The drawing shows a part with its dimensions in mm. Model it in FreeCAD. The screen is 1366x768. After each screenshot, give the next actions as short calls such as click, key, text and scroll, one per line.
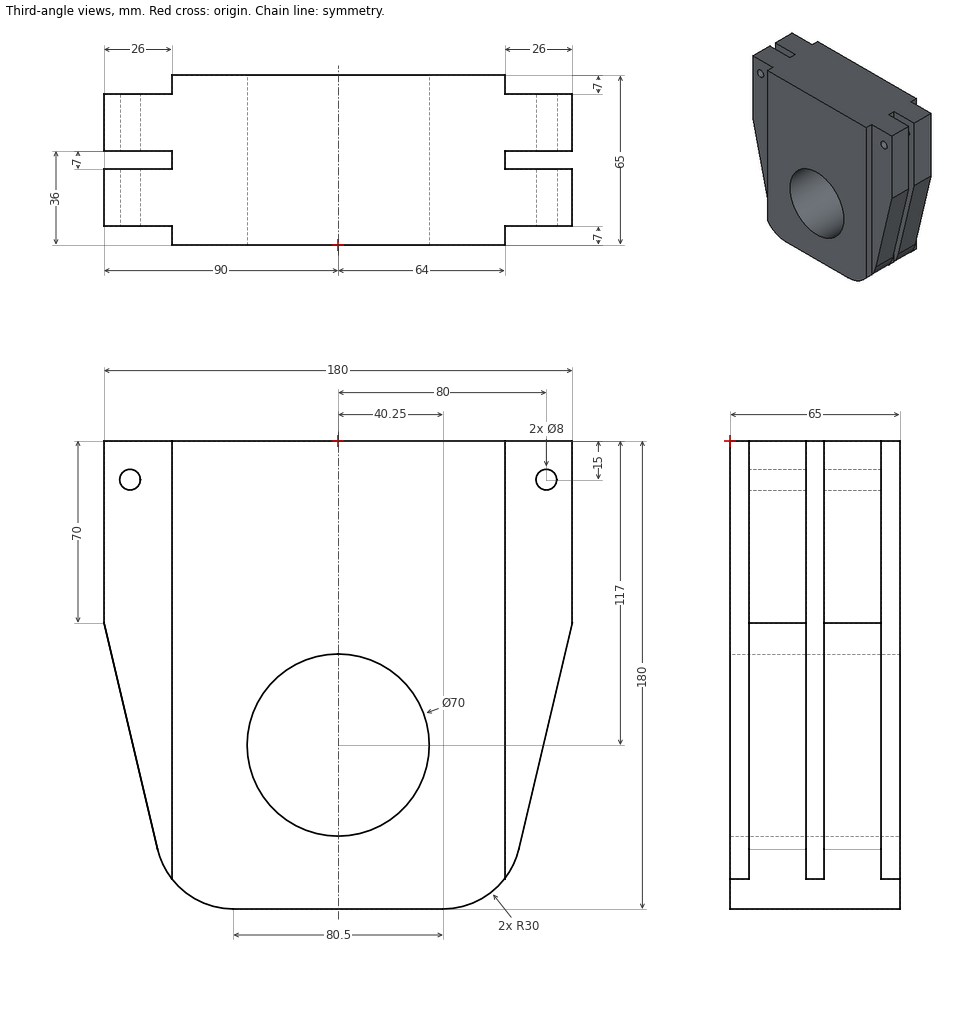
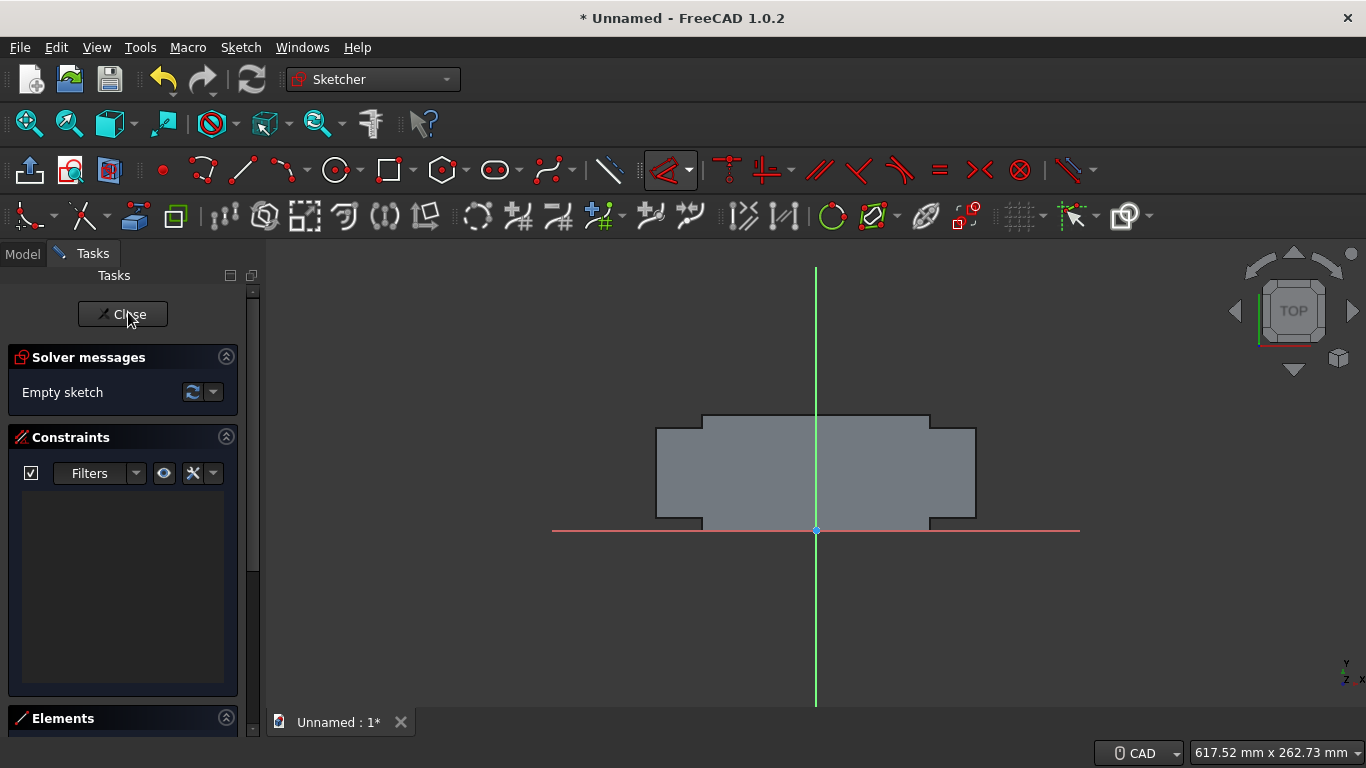
scroll(899, 530, up, 3)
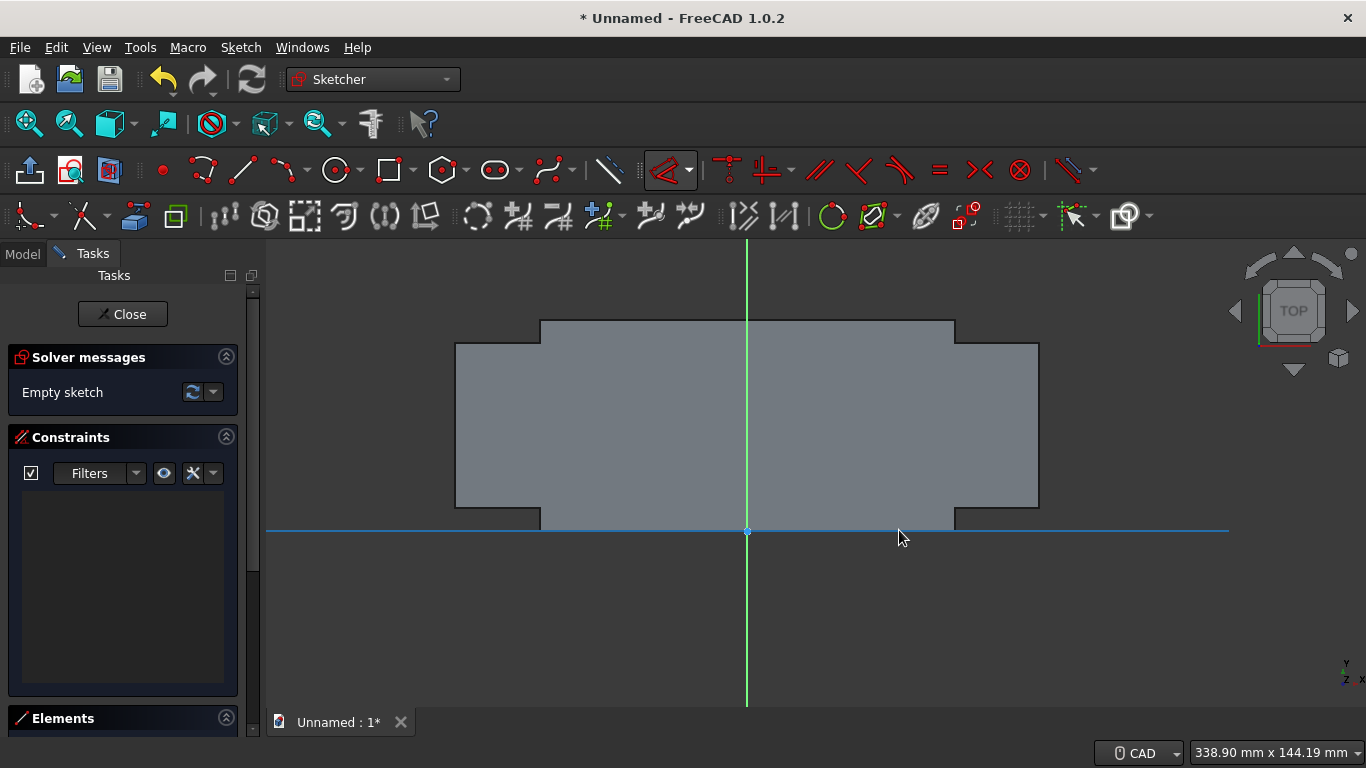
click(390, 170)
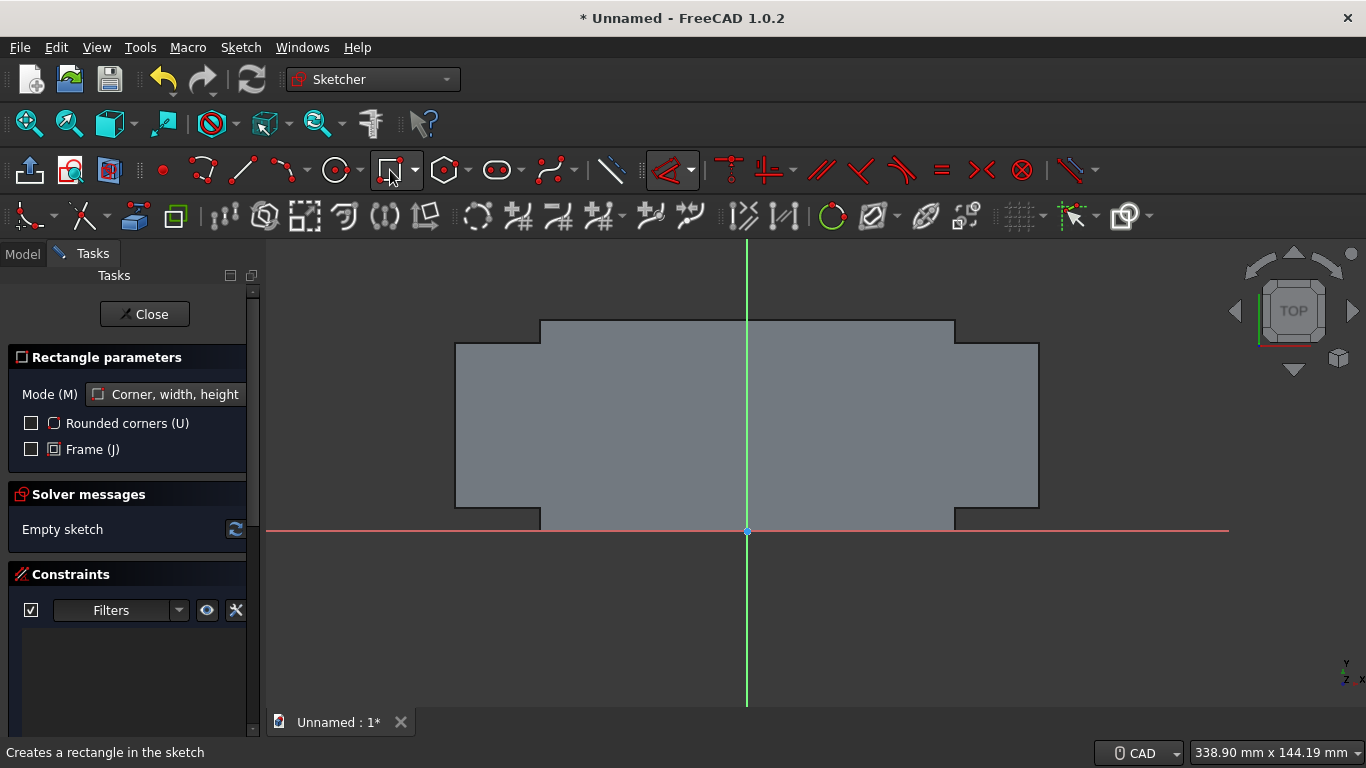
click(455, 414)
move(540, 437)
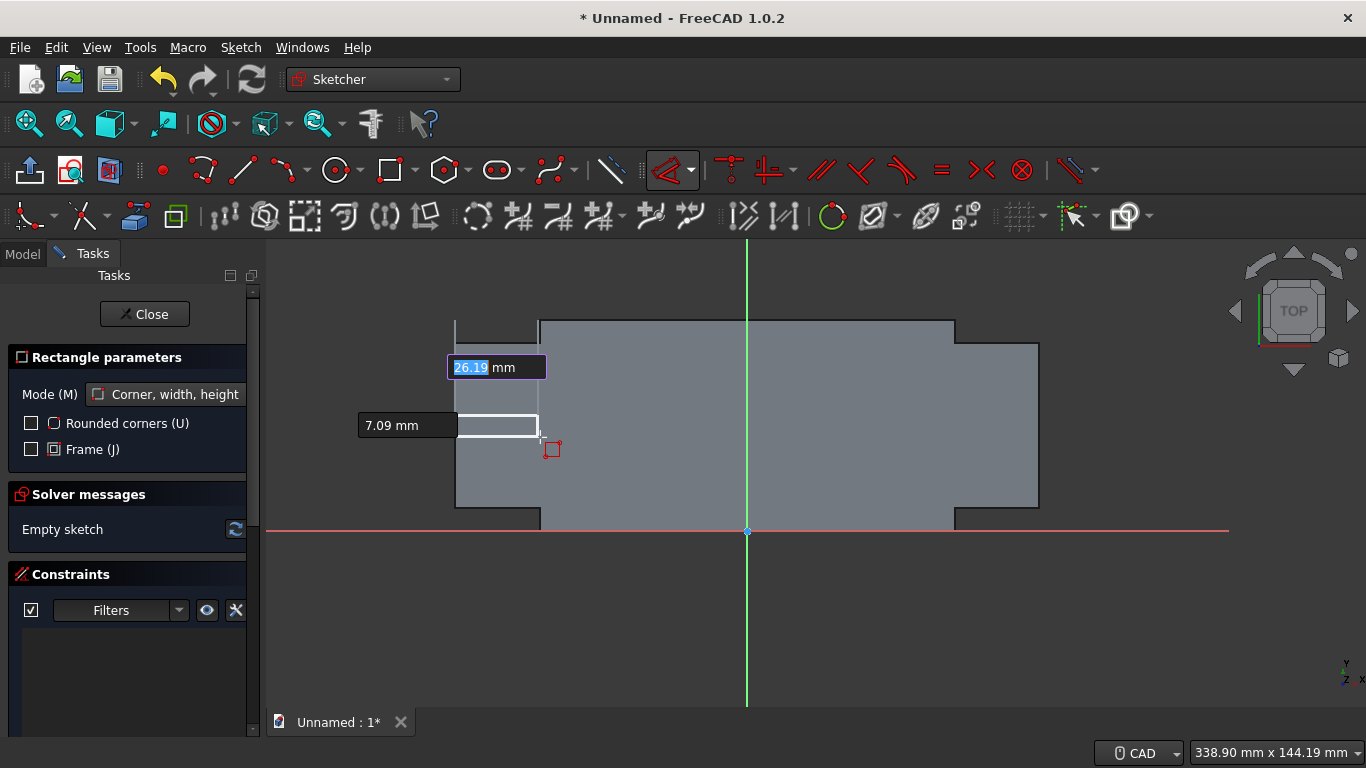
text(26)
key(Tab)
text(7)
key(Return)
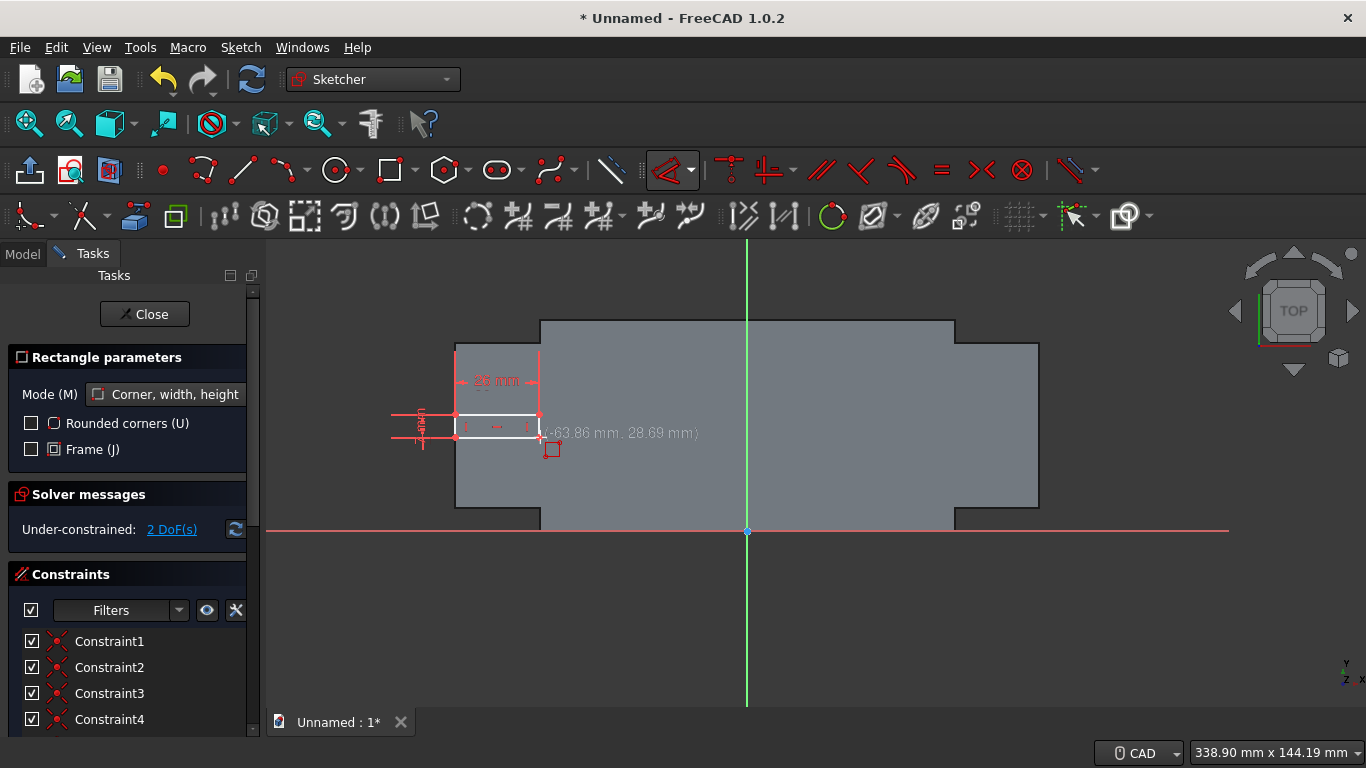
click(955, 414)
move(1039, 437)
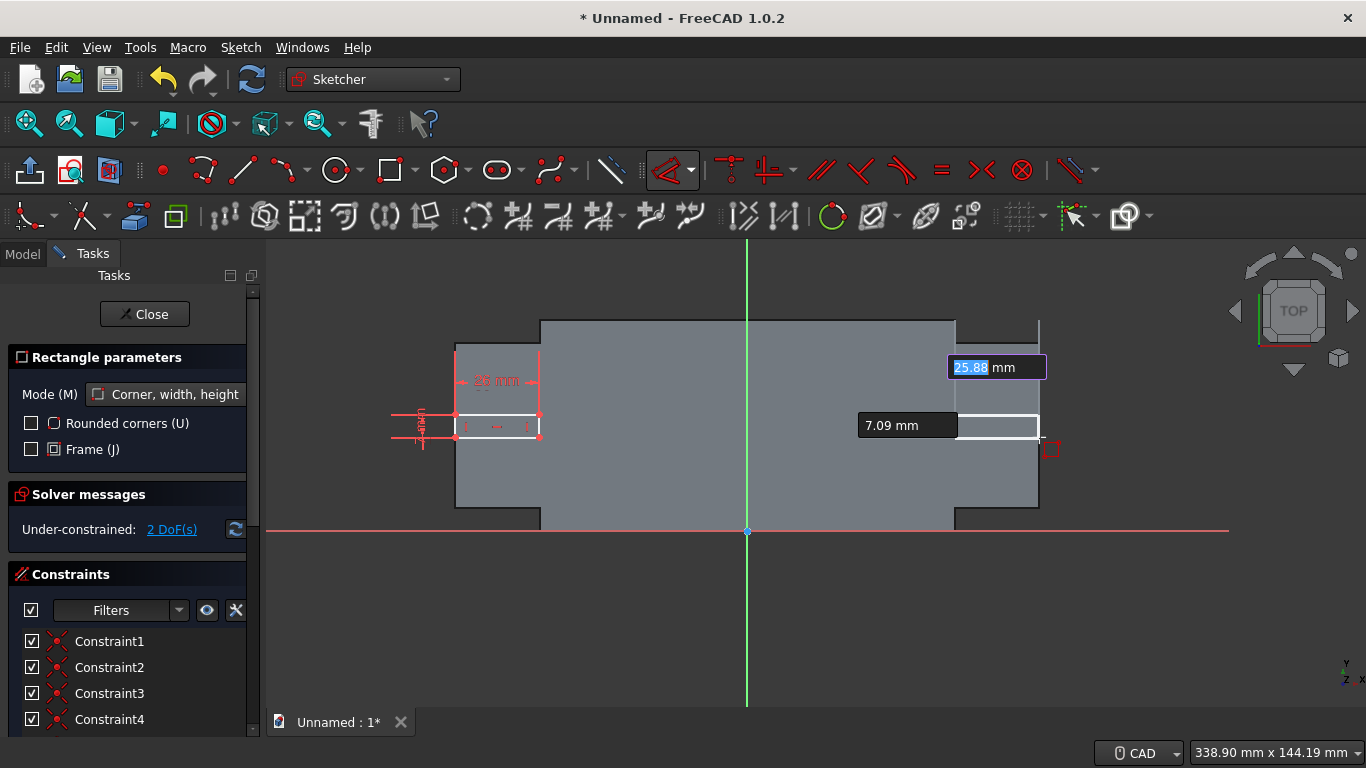
text(26)
key(Tab)
text(7)
key(Return)
key(Escape)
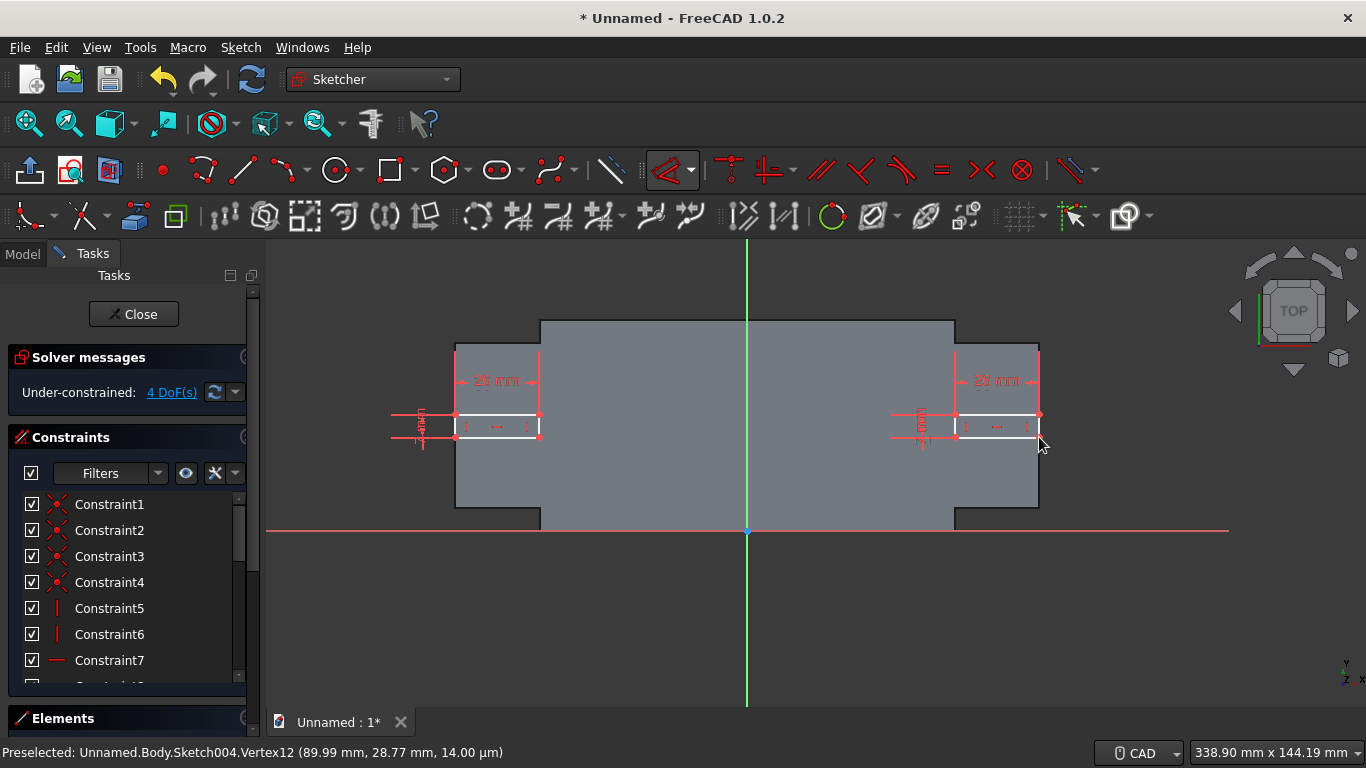
click(539, 415)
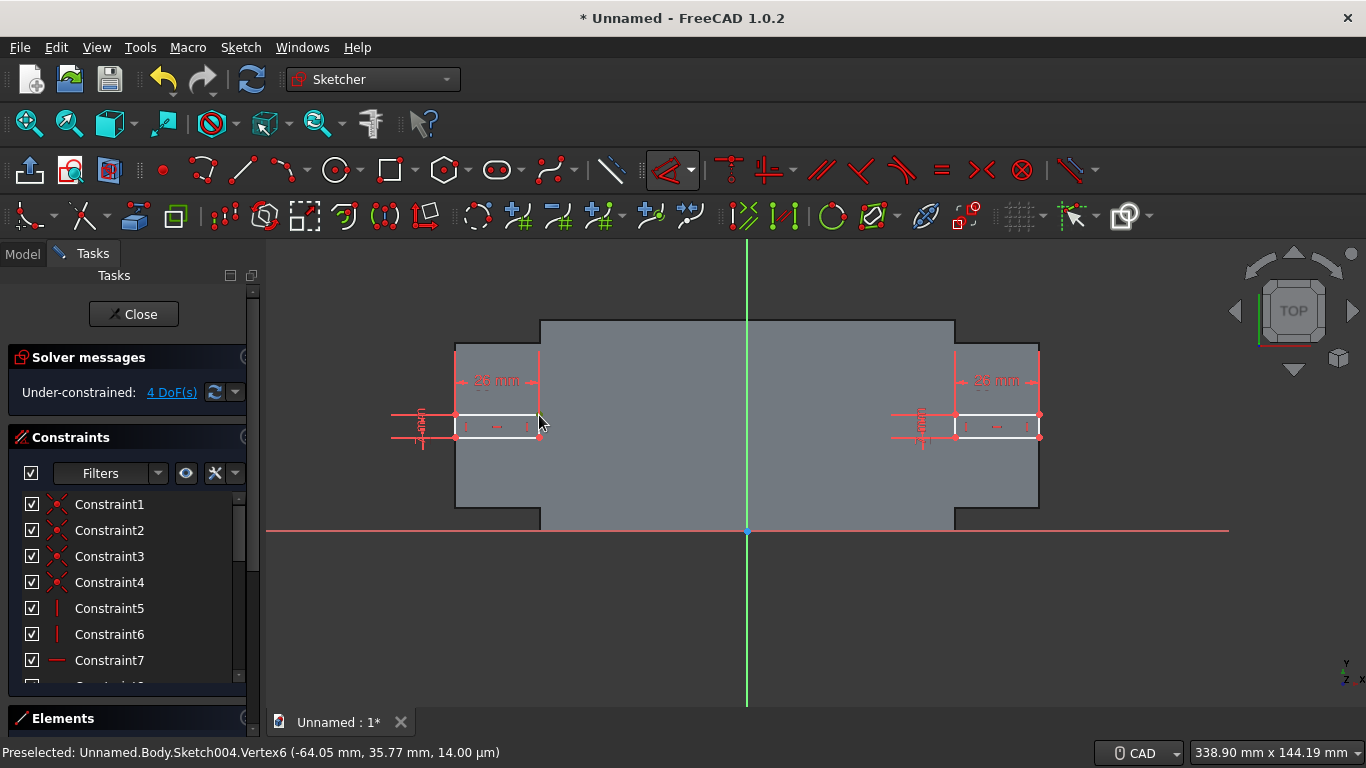
click(955, 415)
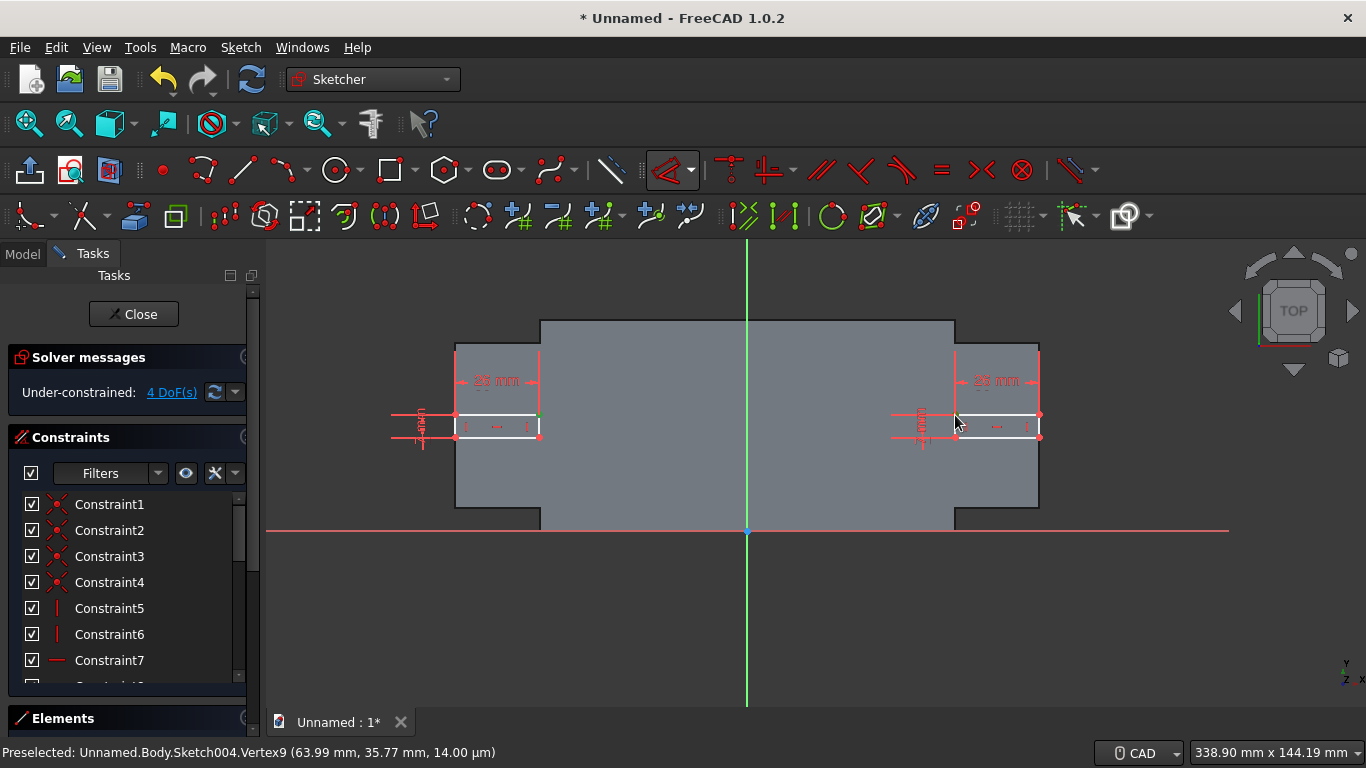
click(747, 650)